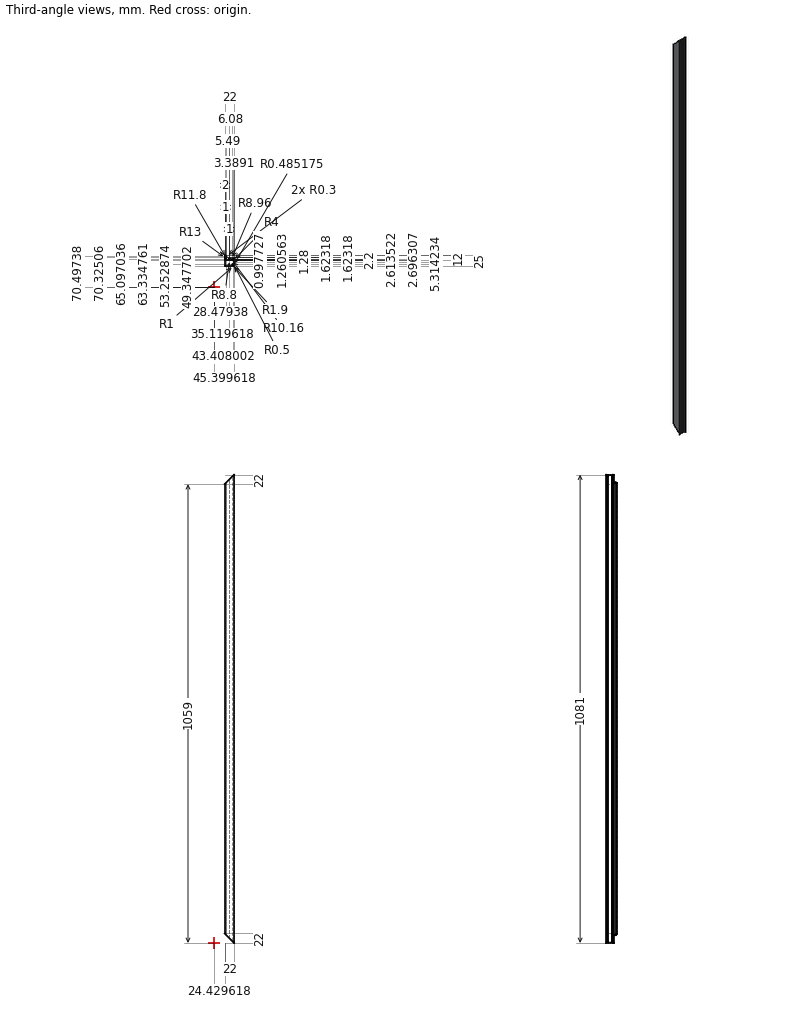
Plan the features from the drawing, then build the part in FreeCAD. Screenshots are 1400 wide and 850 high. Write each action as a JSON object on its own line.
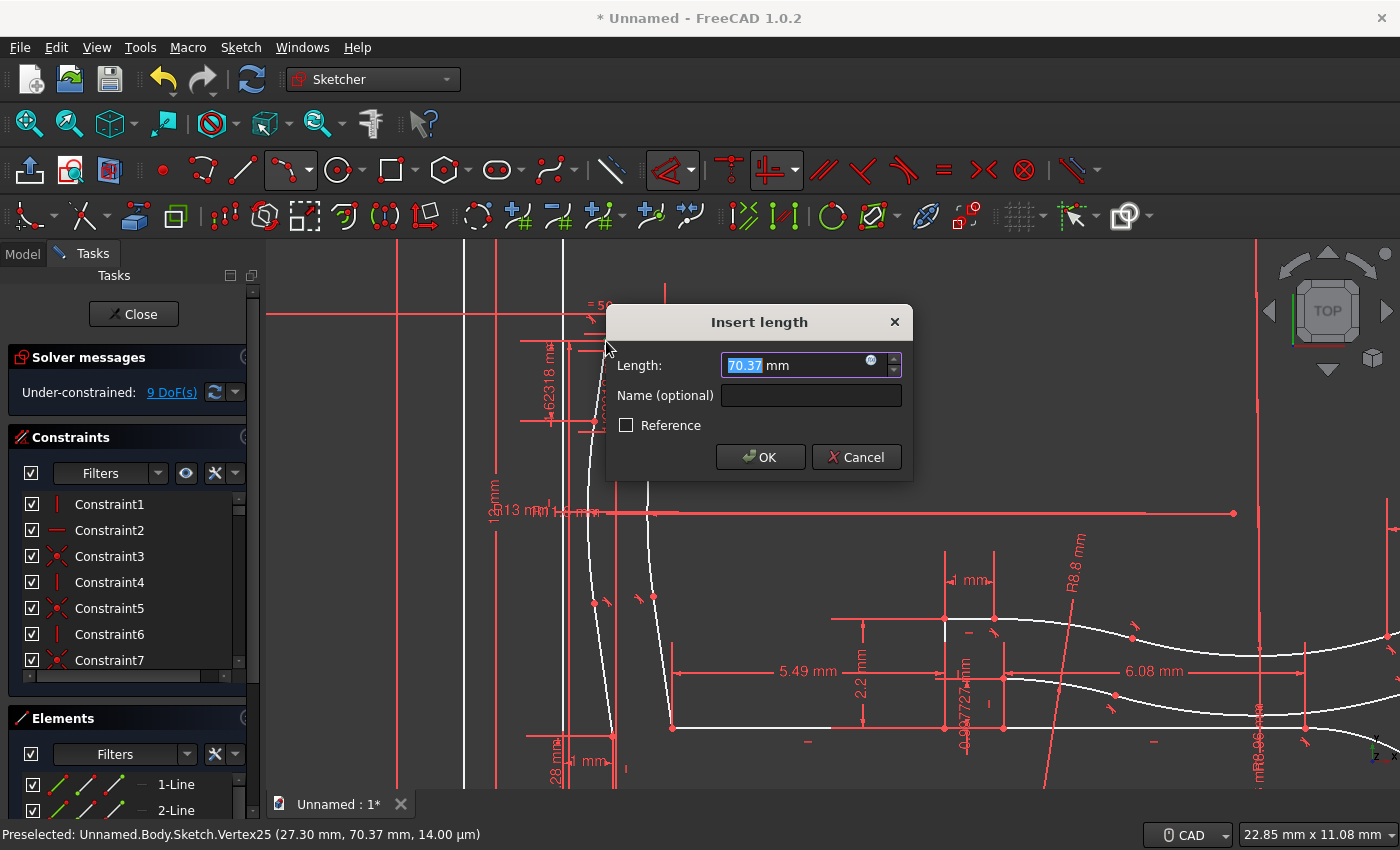
{"action": "type", "text": "70.32506"}
{"action": "key", "text": "Return"}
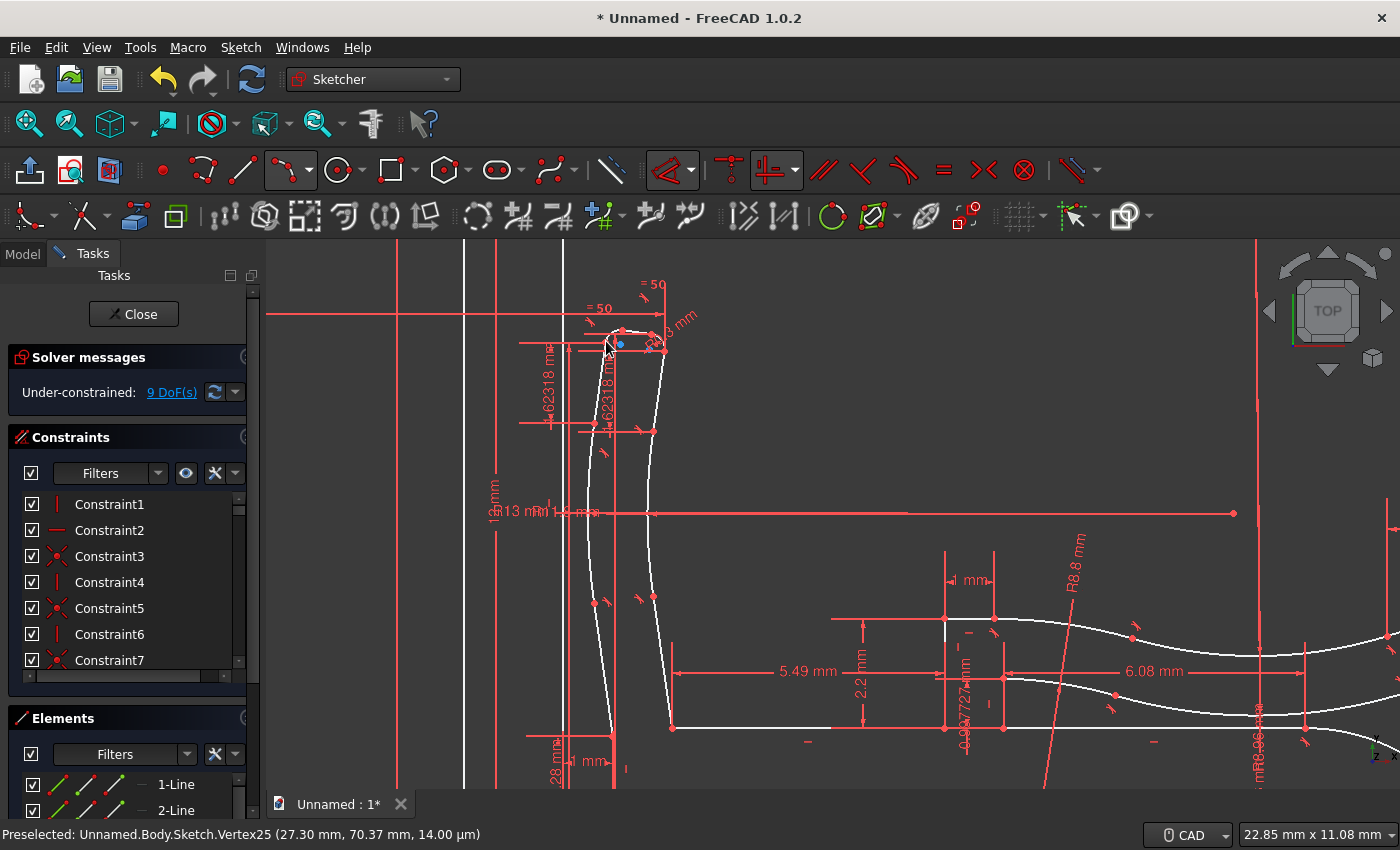
{"action": "left_click", "coordinate": [666, 689]}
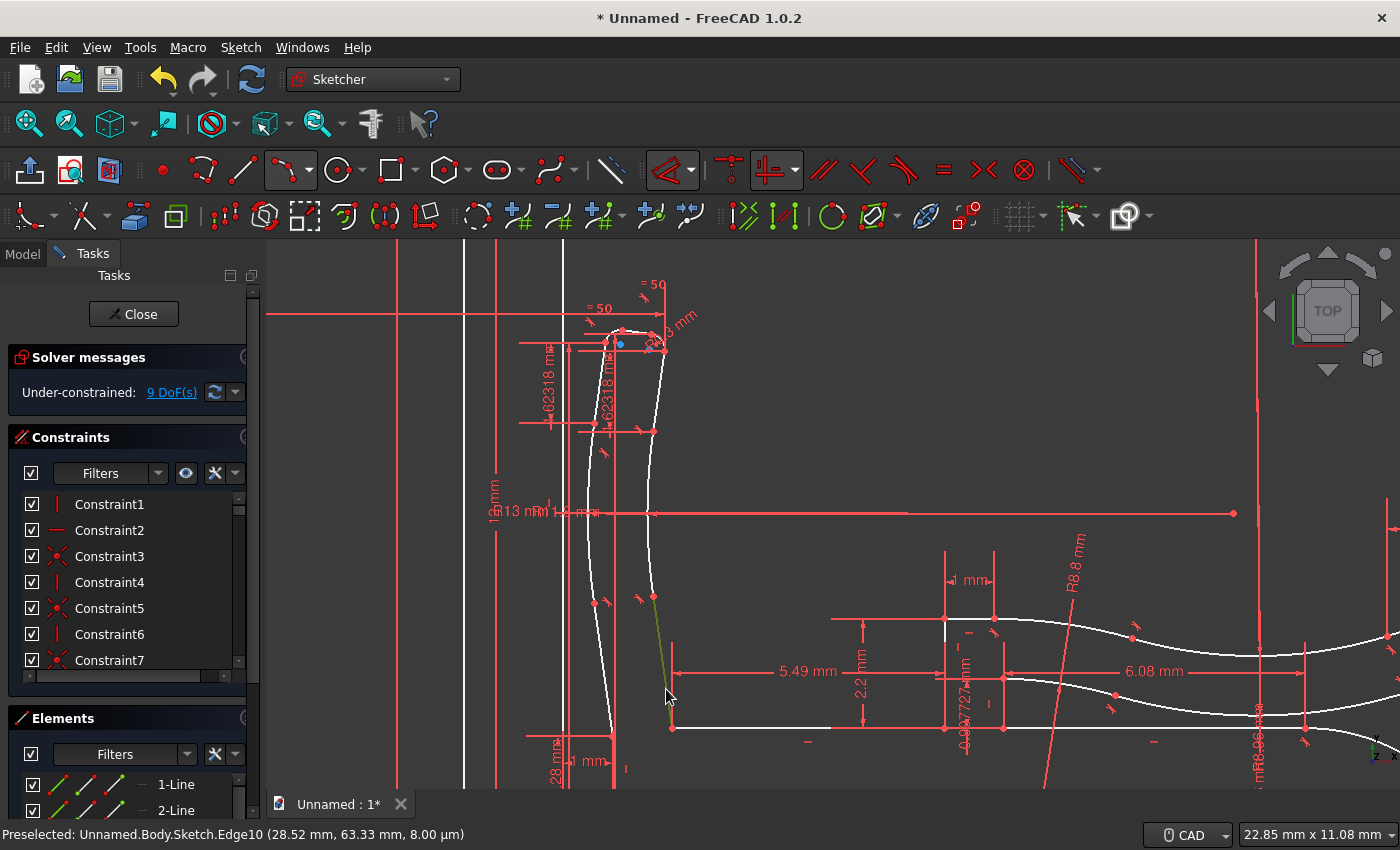
{"action": "left_click", "coordinate": [694, 170]}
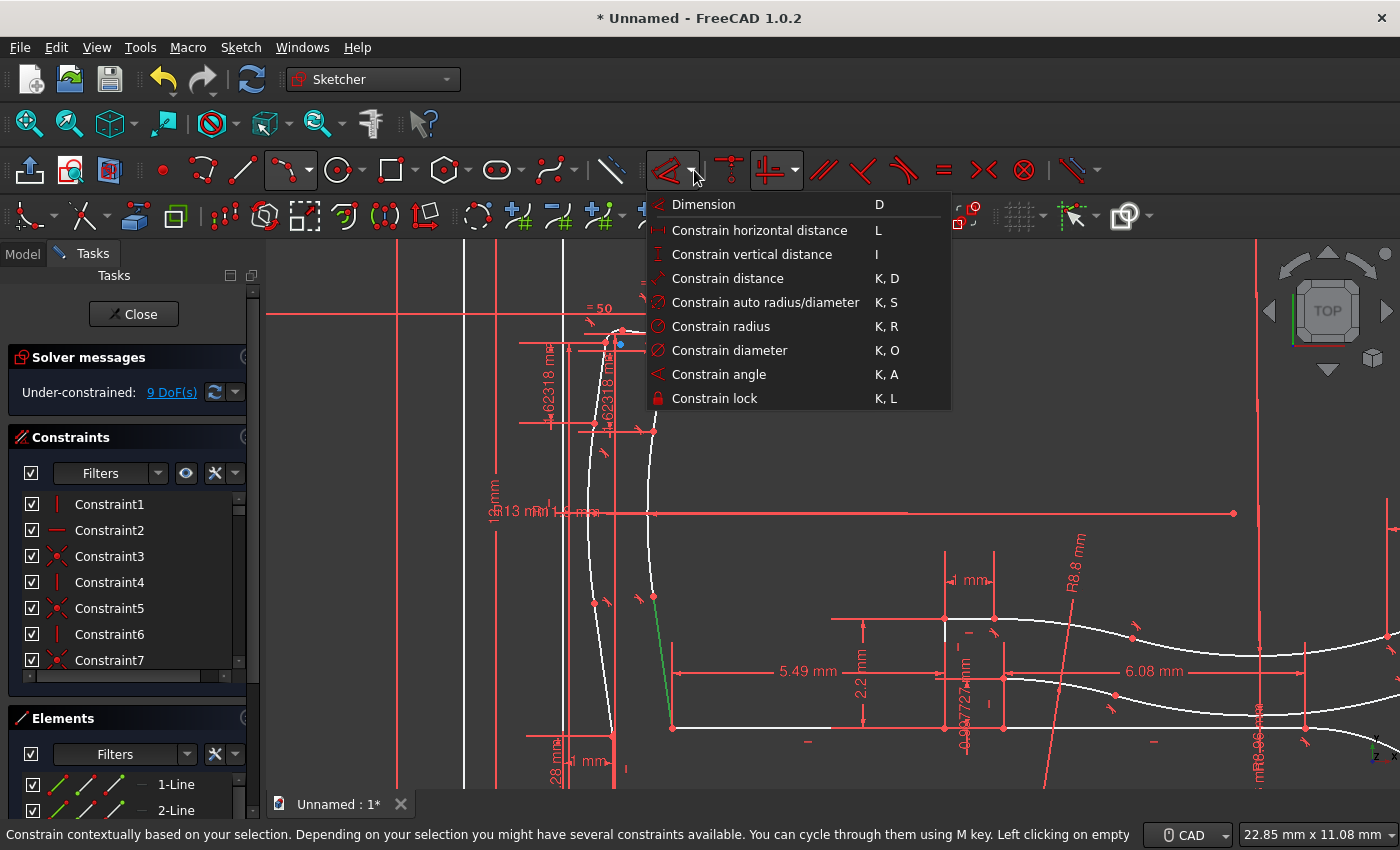
{"action": "left_click", "coordinate": [799, 254]}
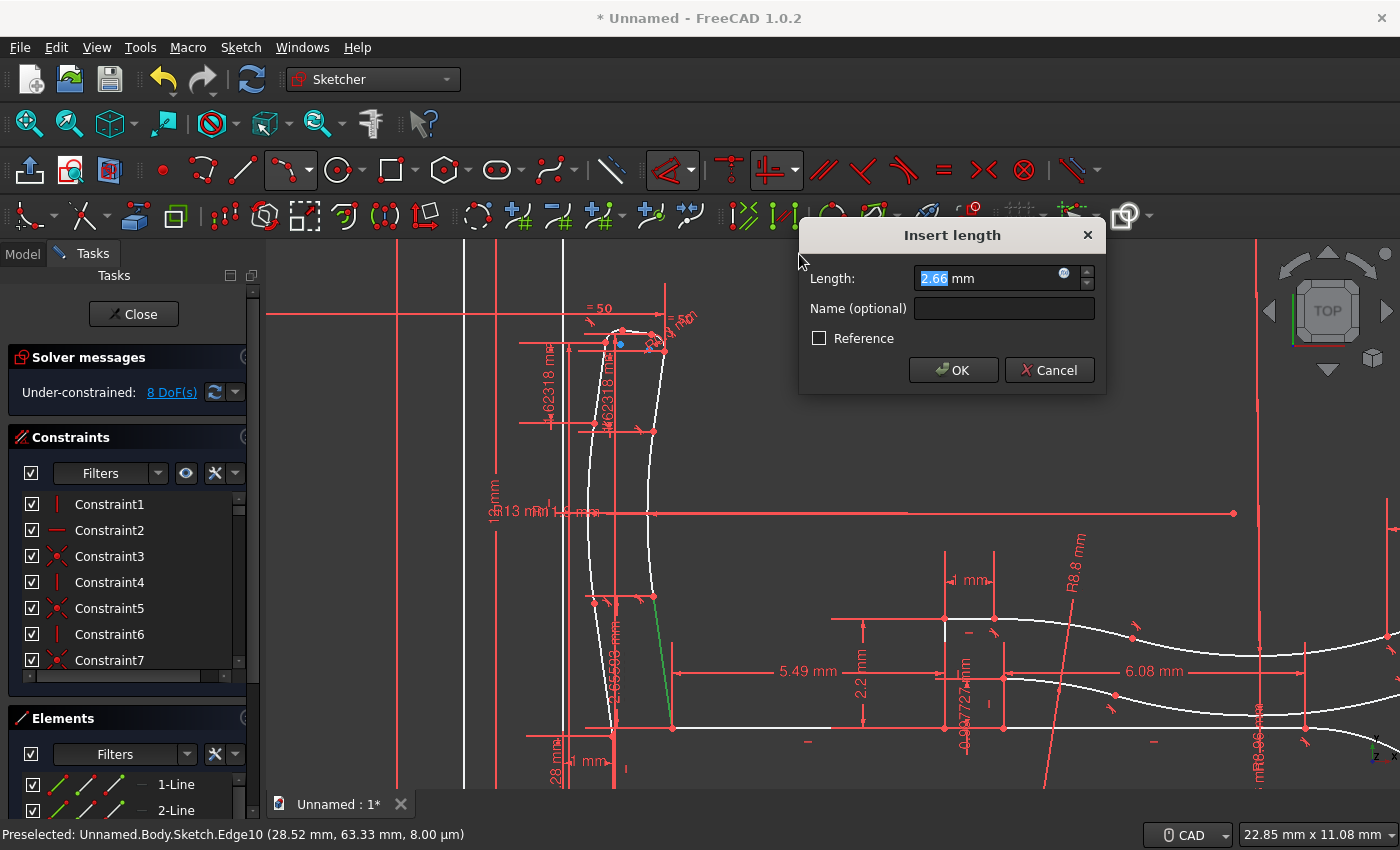
{"action": "type", "text": "2.696307"}
{"action": "key", "text": "Return"}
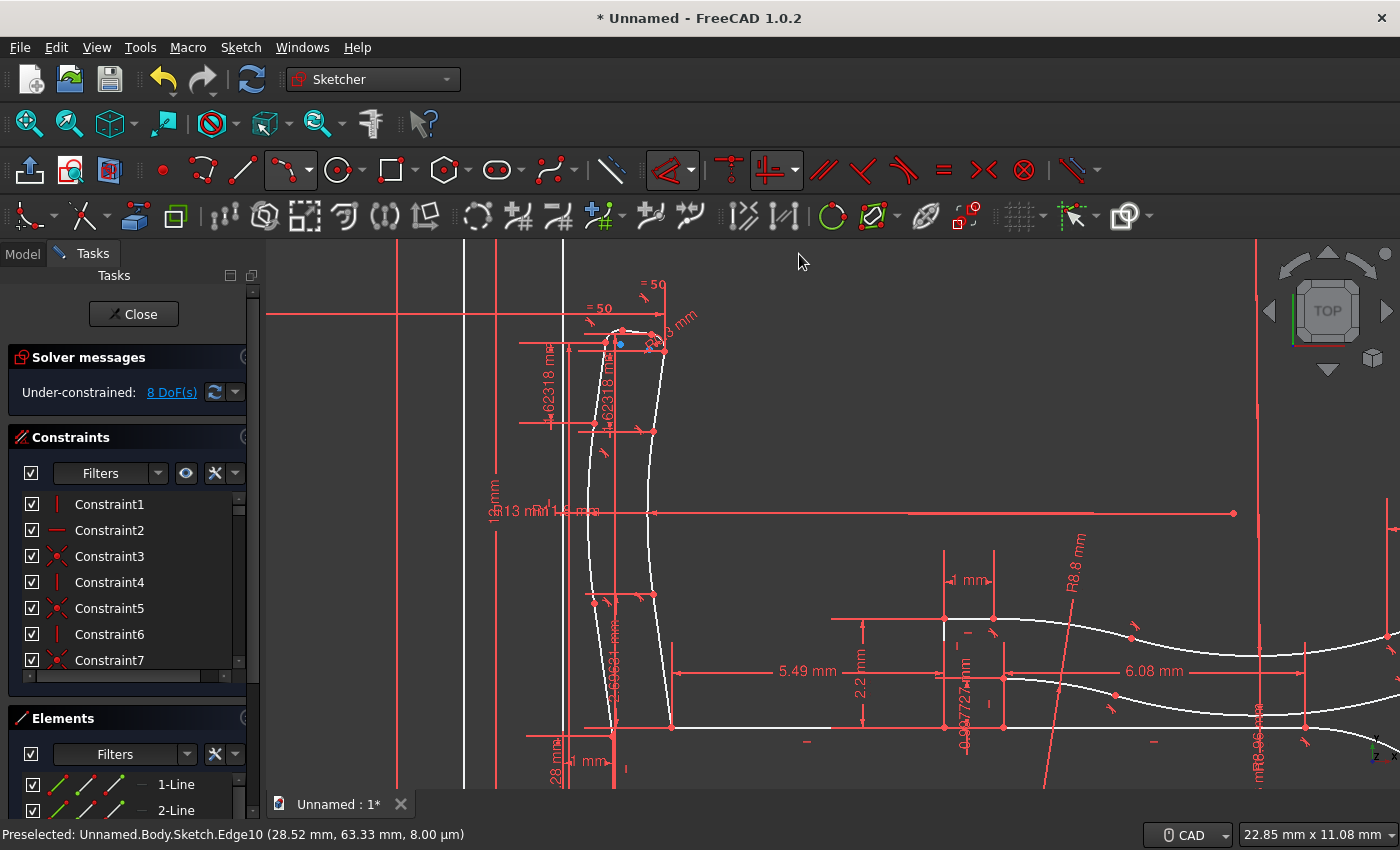
{"action": "left_click", "coordinate": [600, 643]}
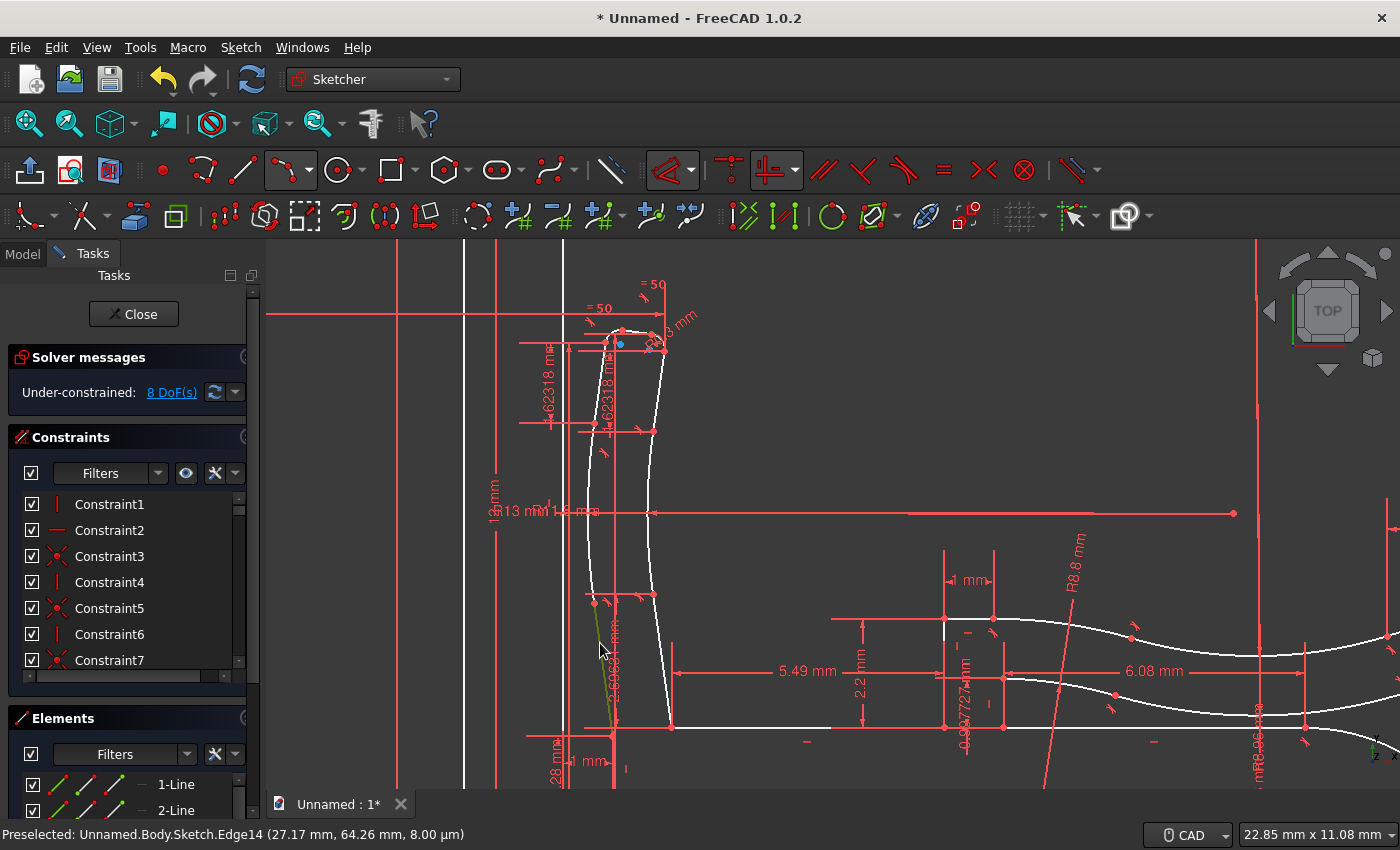
{"action": "left_click", "coordinate": [694, 170]}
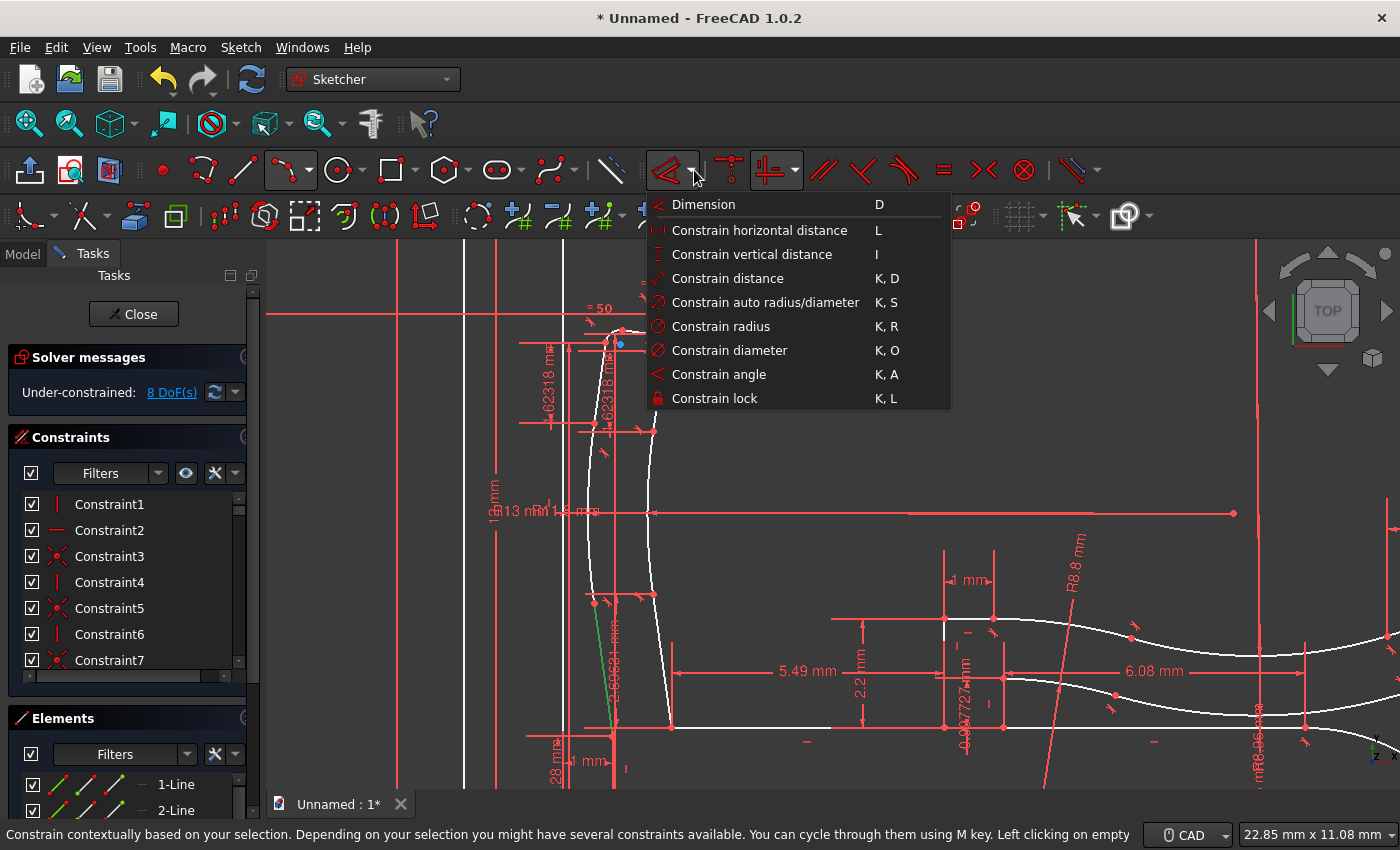
{"action": "left_click", "coordinate": [799, 254]}